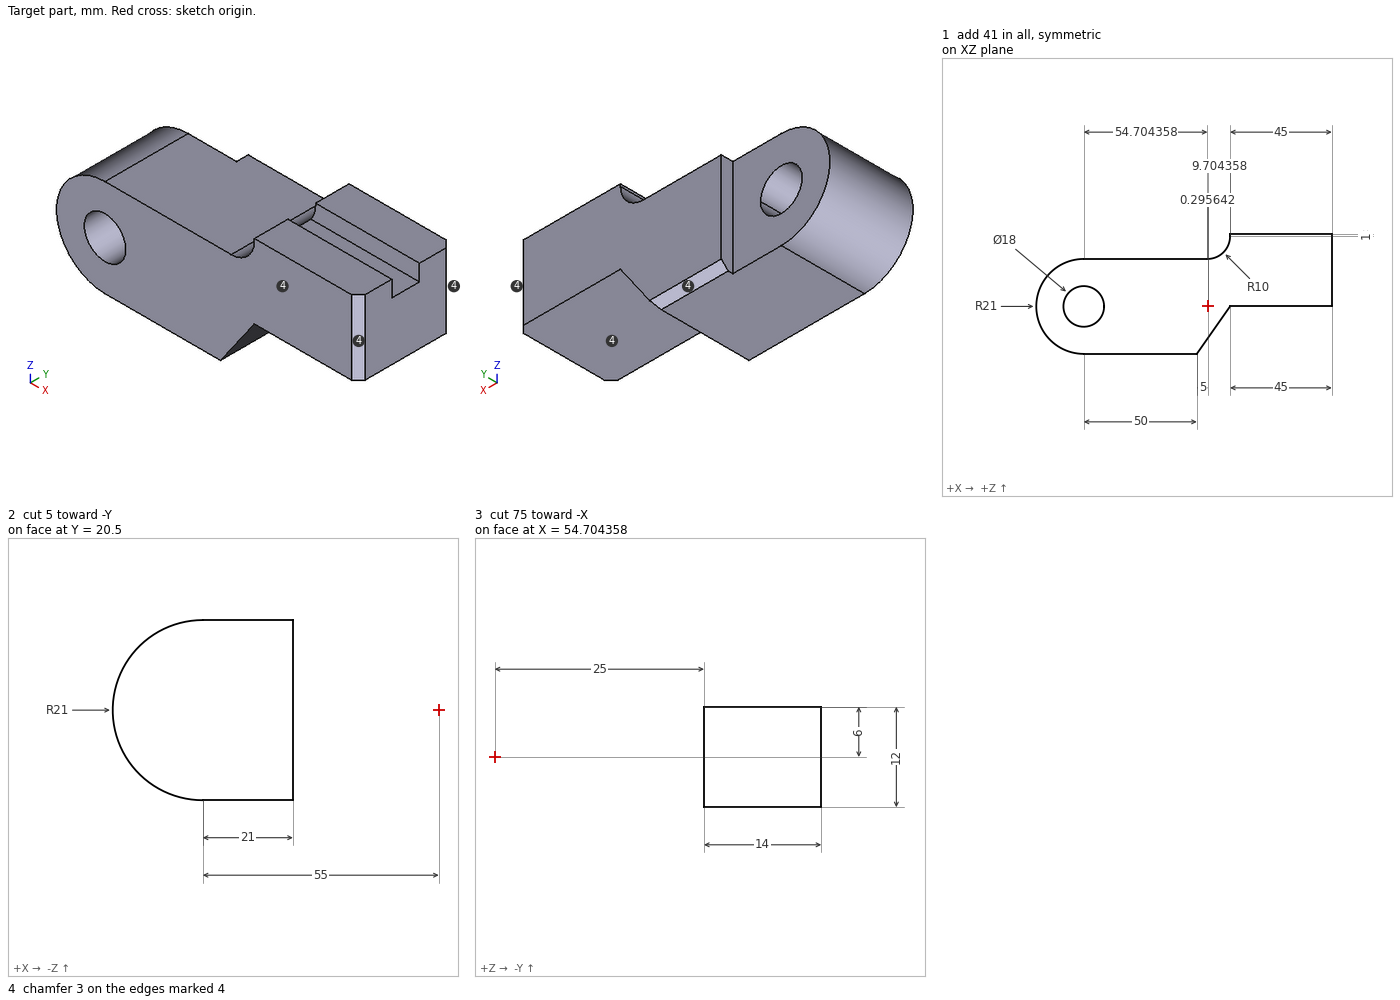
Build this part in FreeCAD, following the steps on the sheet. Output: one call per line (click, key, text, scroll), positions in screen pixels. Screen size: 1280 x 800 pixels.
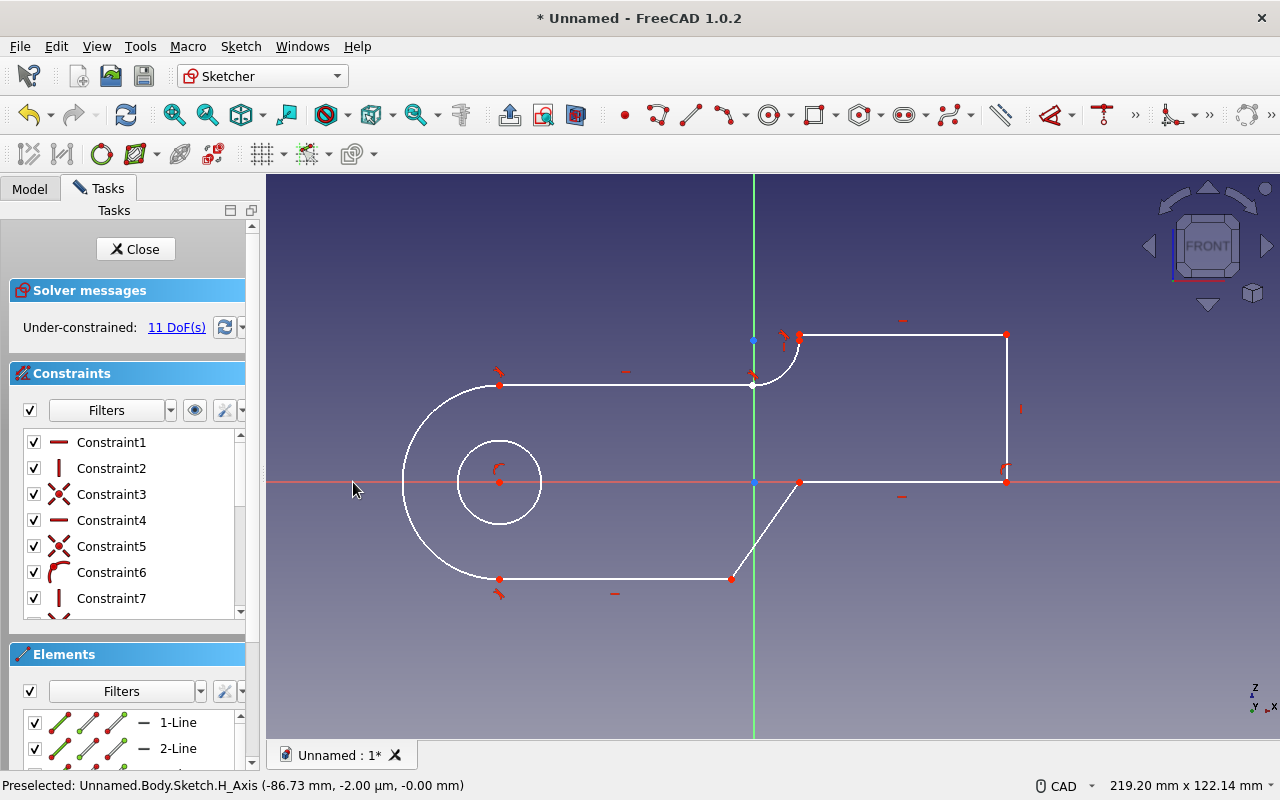
click(1050, 116)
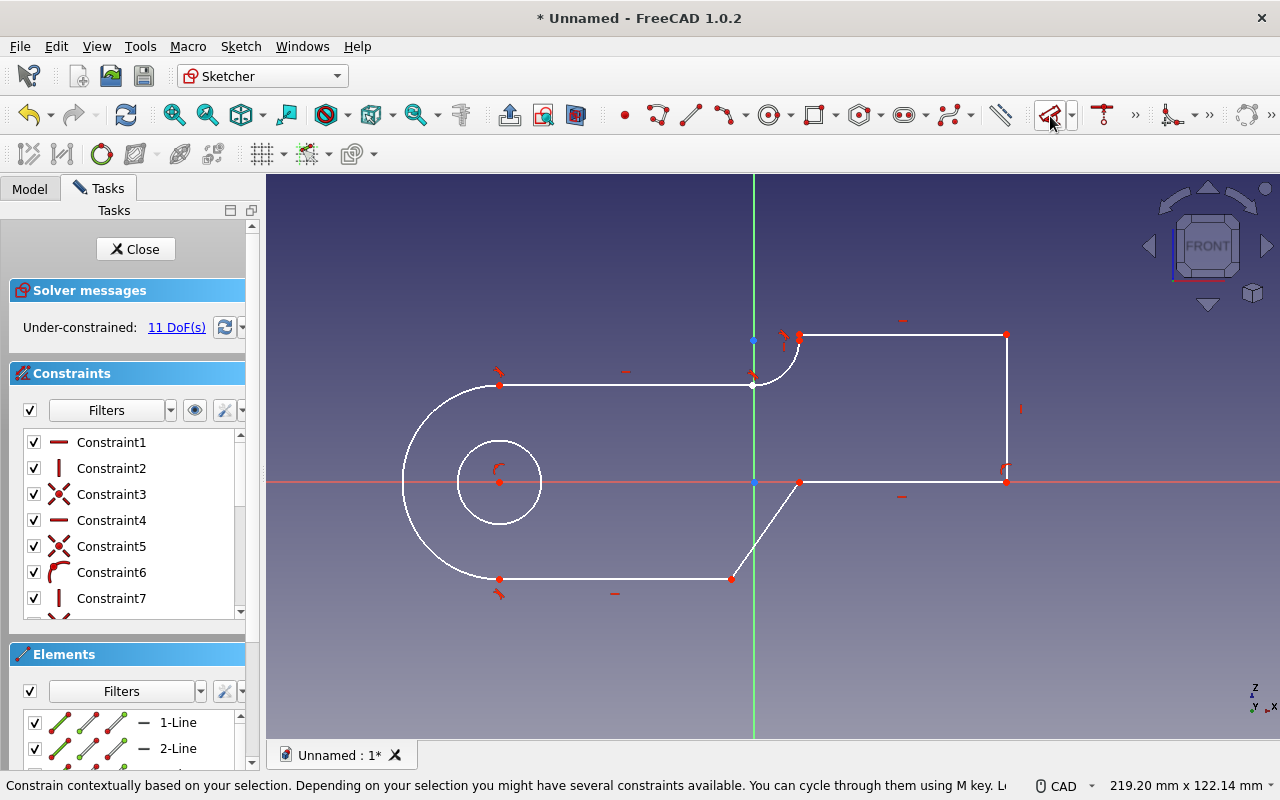
click(774, 381)
click(788, 410)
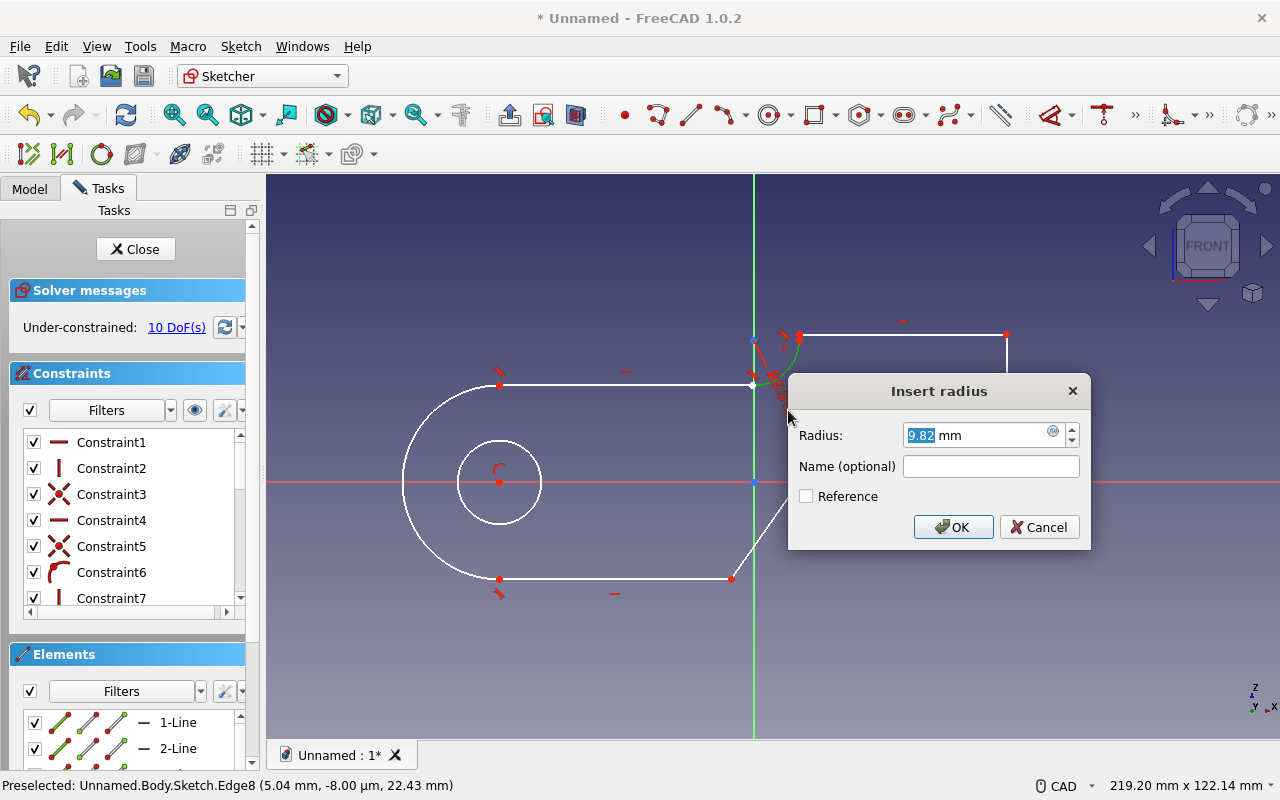
text(10)
key(Return)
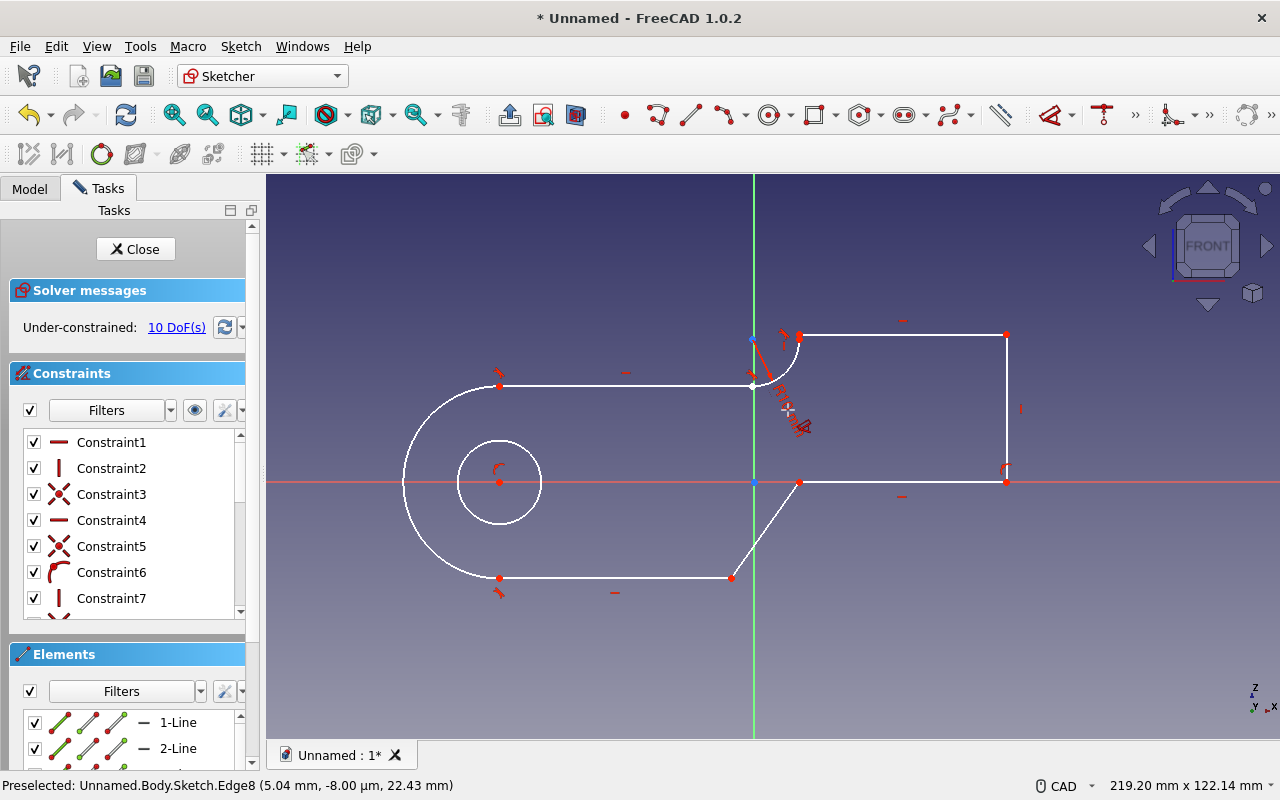
click(422, 426)
click(396, 407)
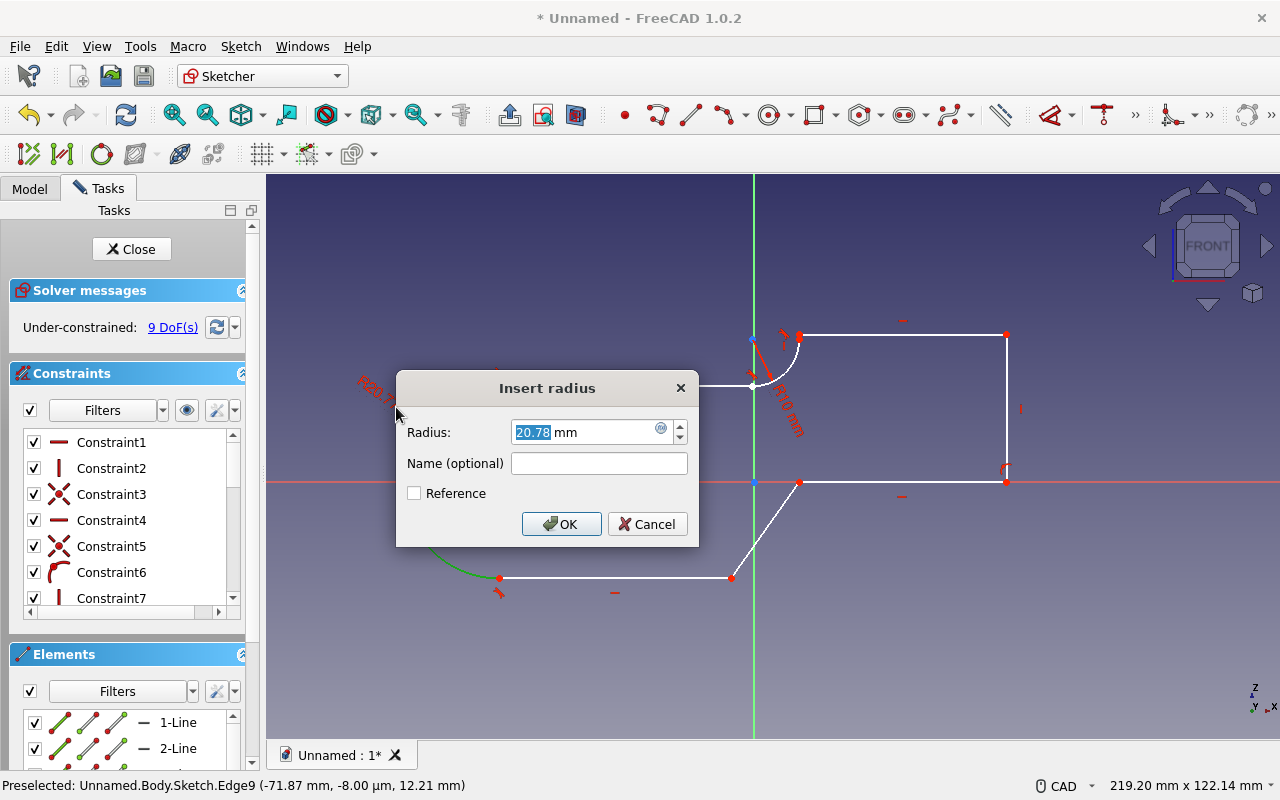
text(21)
key(Return)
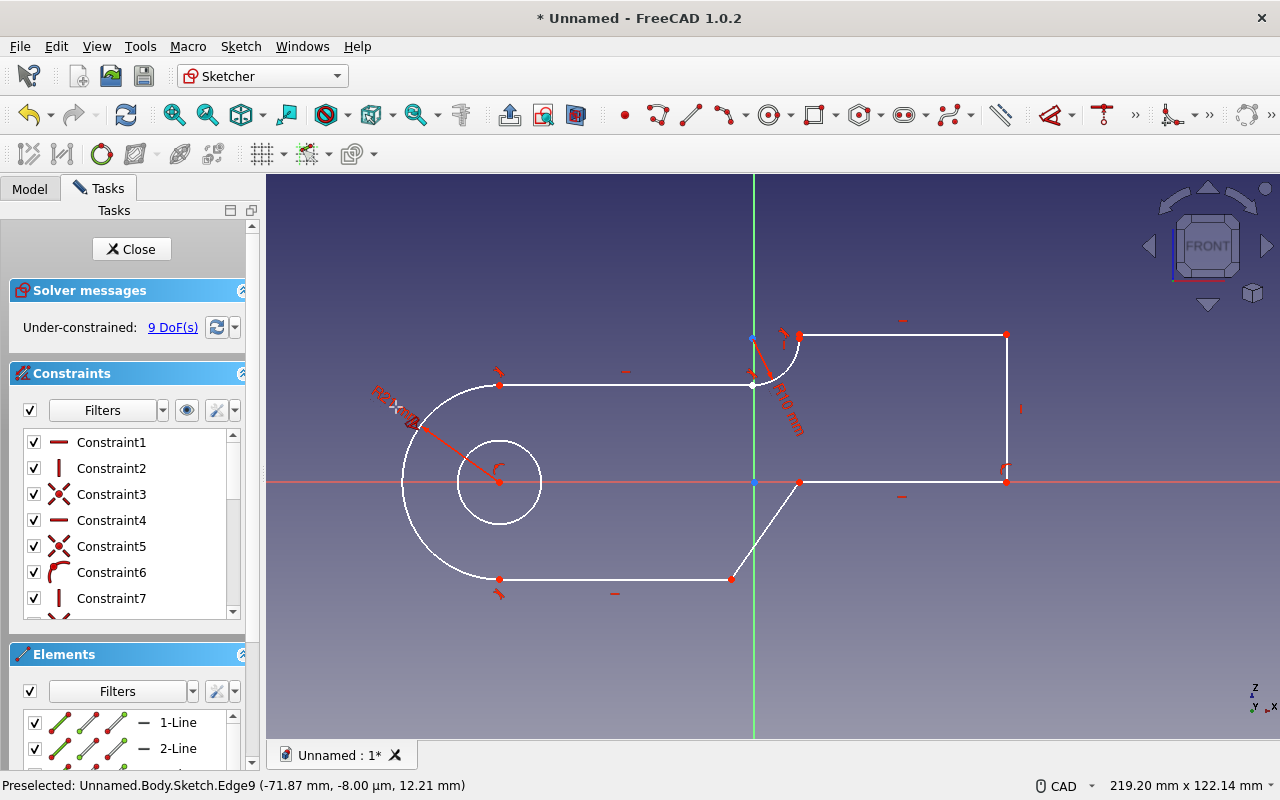
click(529, 453)
click(552, 430)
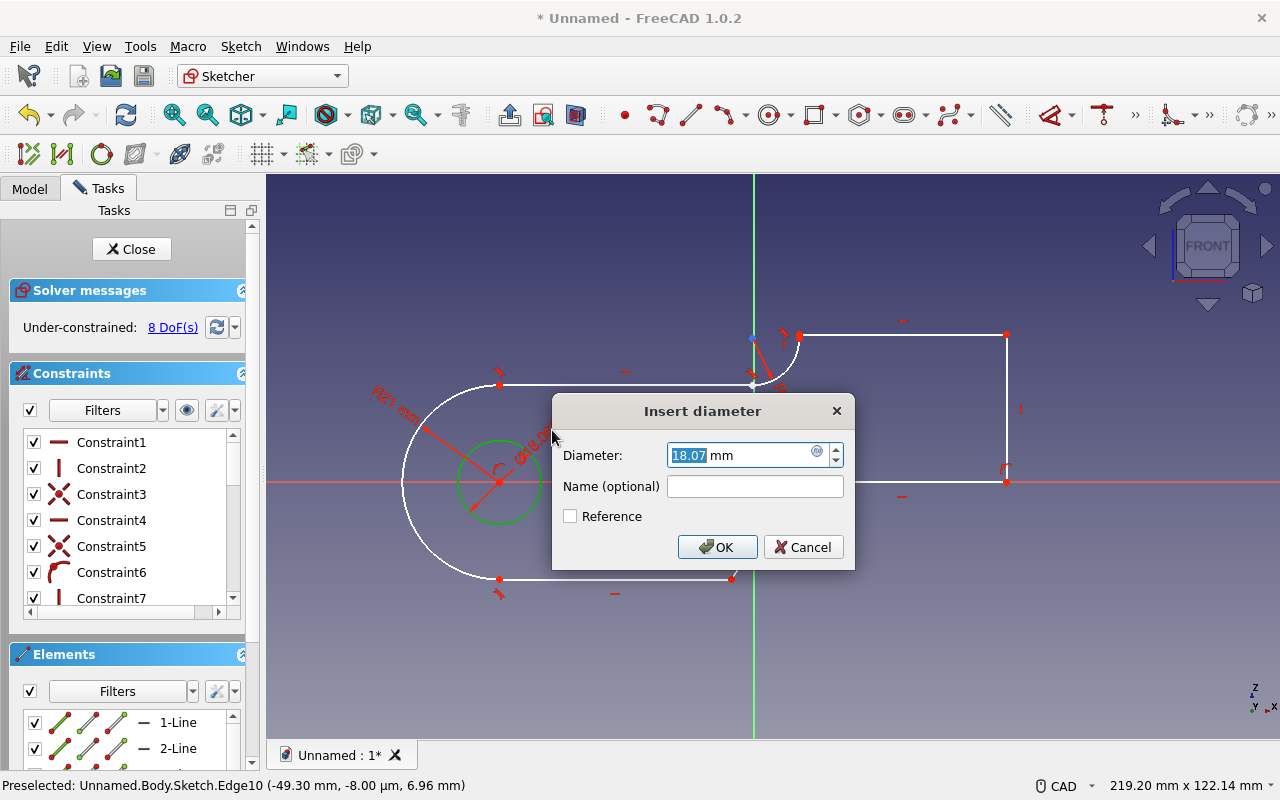
text(18)
key(Return)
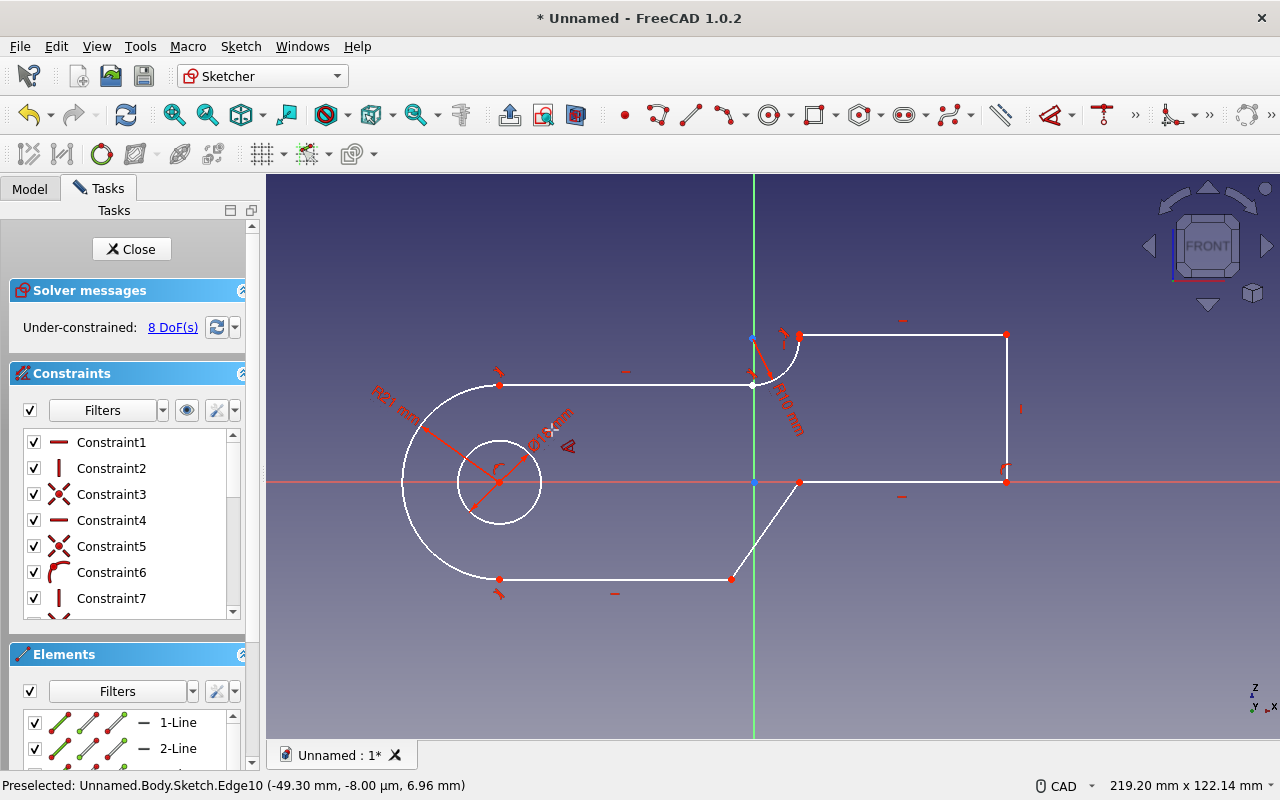
scroll(799, 337, up, 11)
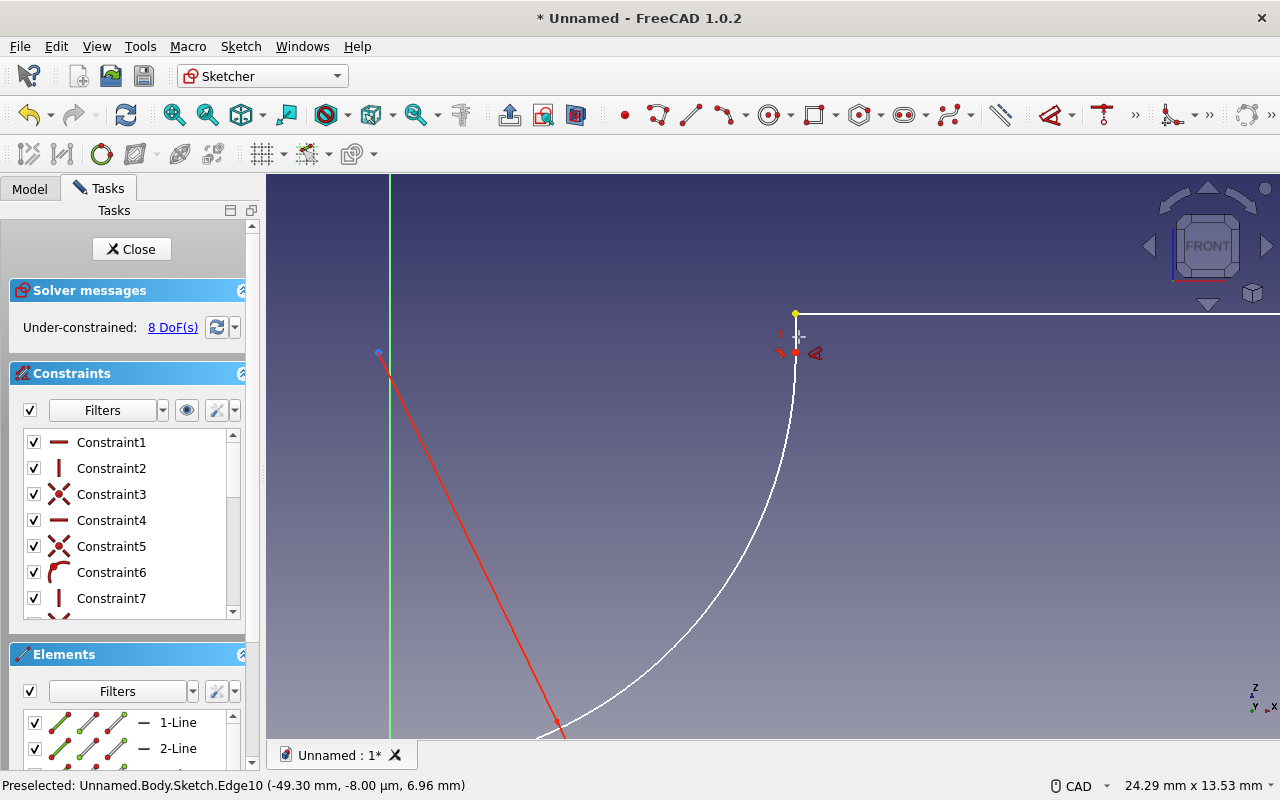
click(796, 333)
click(830, 333)